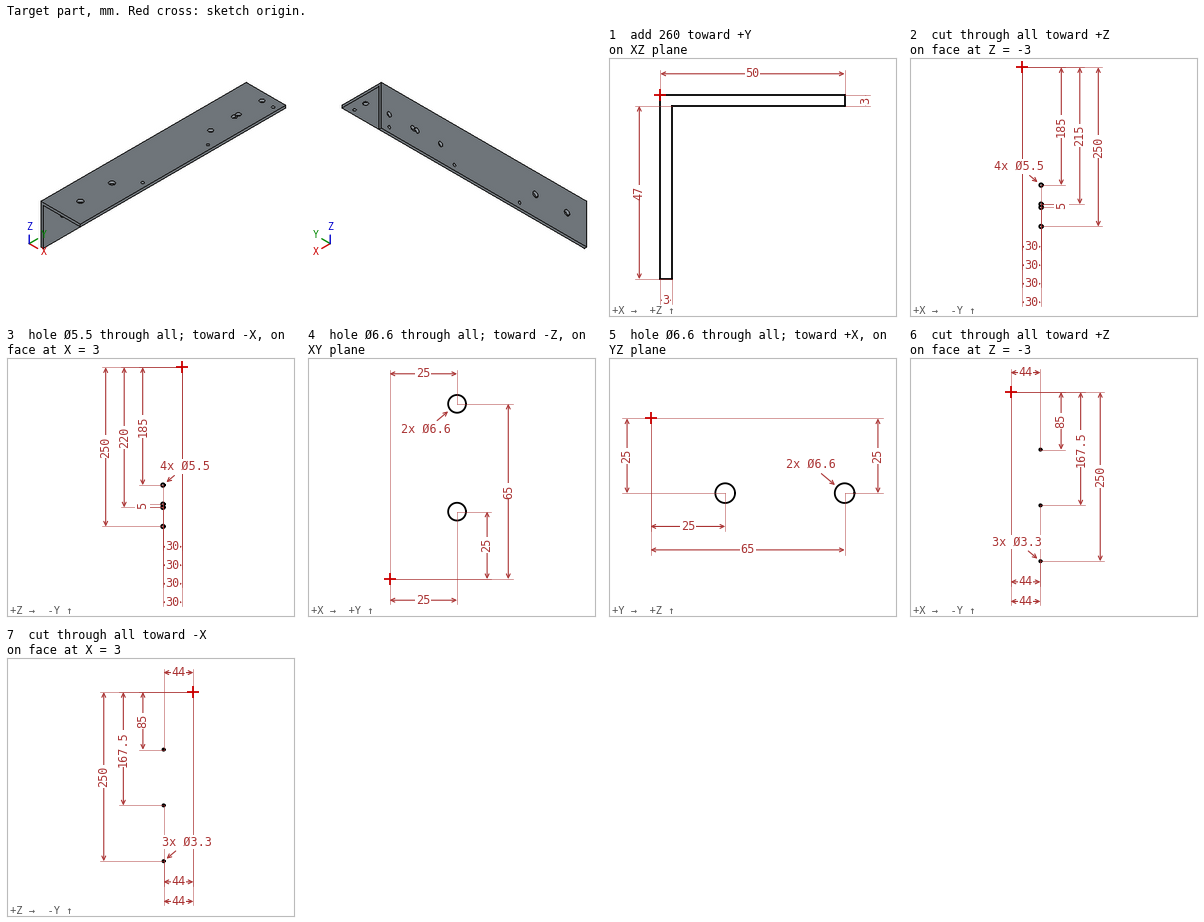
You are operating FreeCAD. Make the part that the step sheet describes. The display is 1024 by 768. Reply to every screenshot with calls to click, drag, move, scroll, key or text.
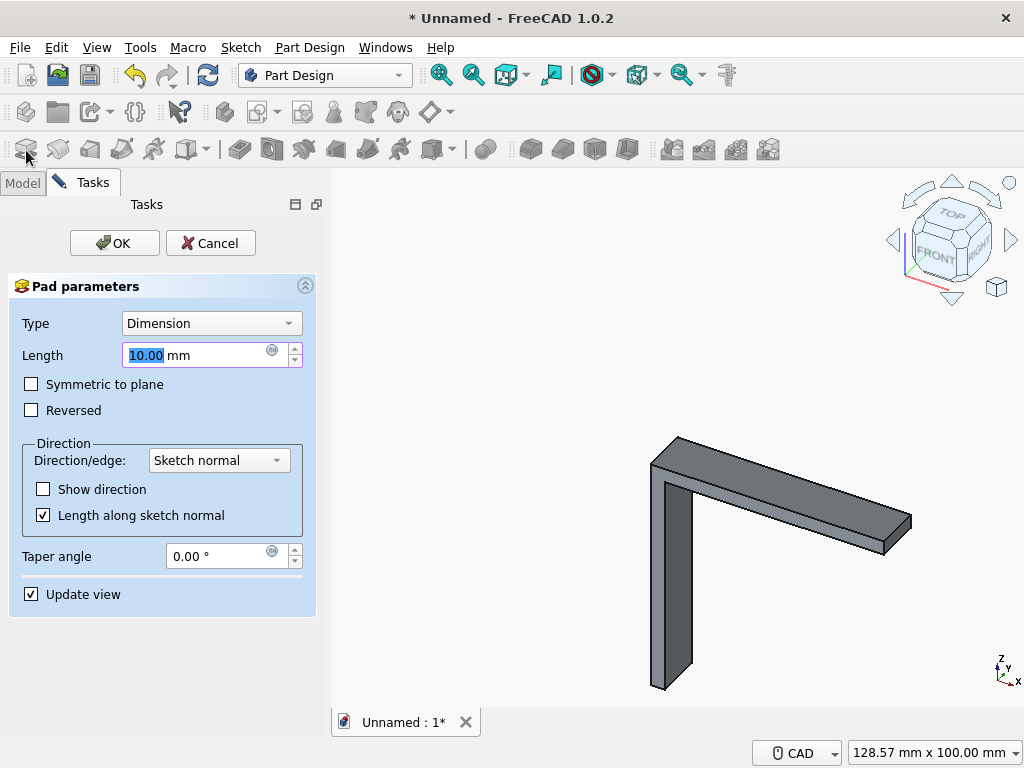
text(260)
key(Tab)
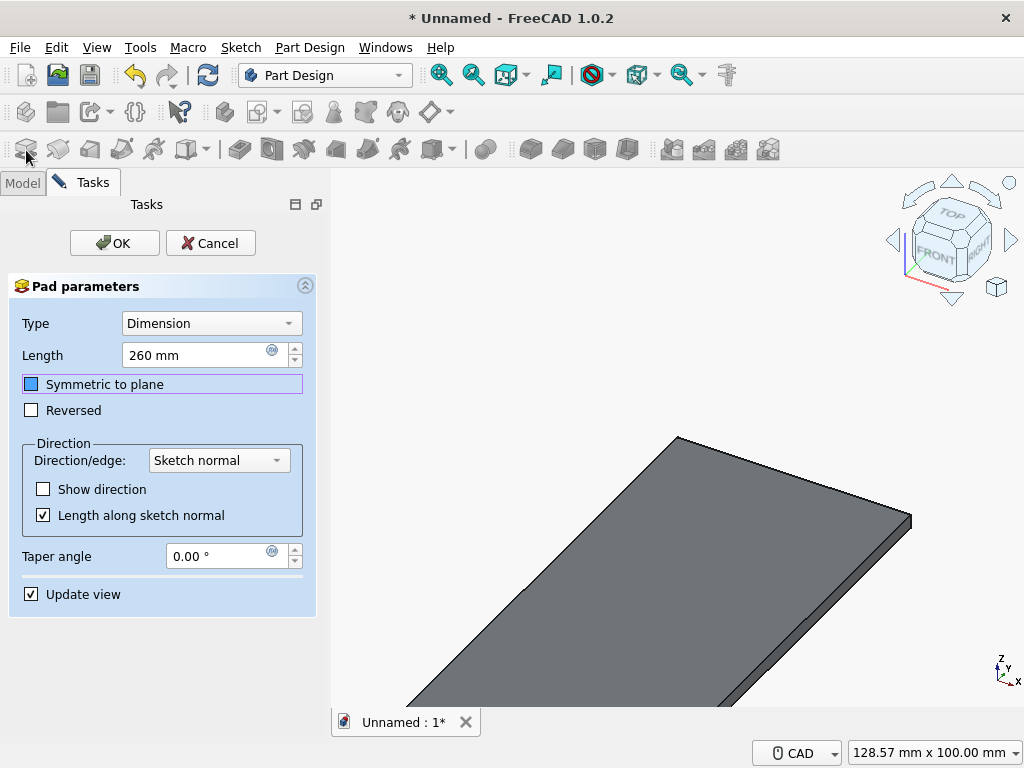
click(30, 410)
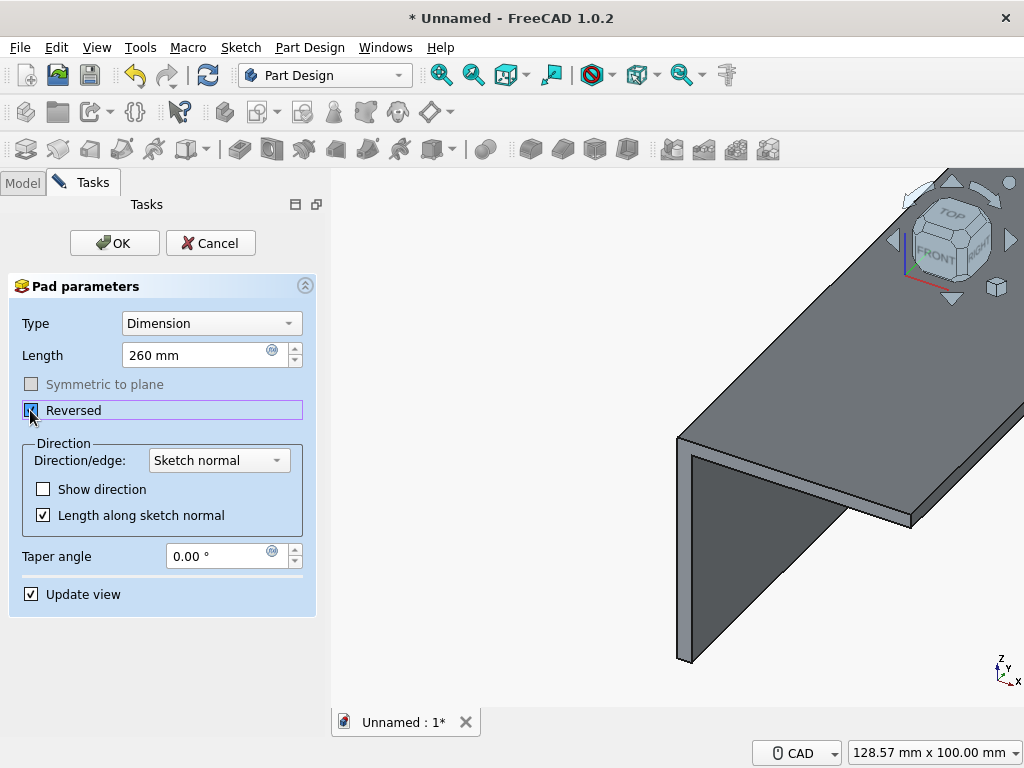
click(115, 243)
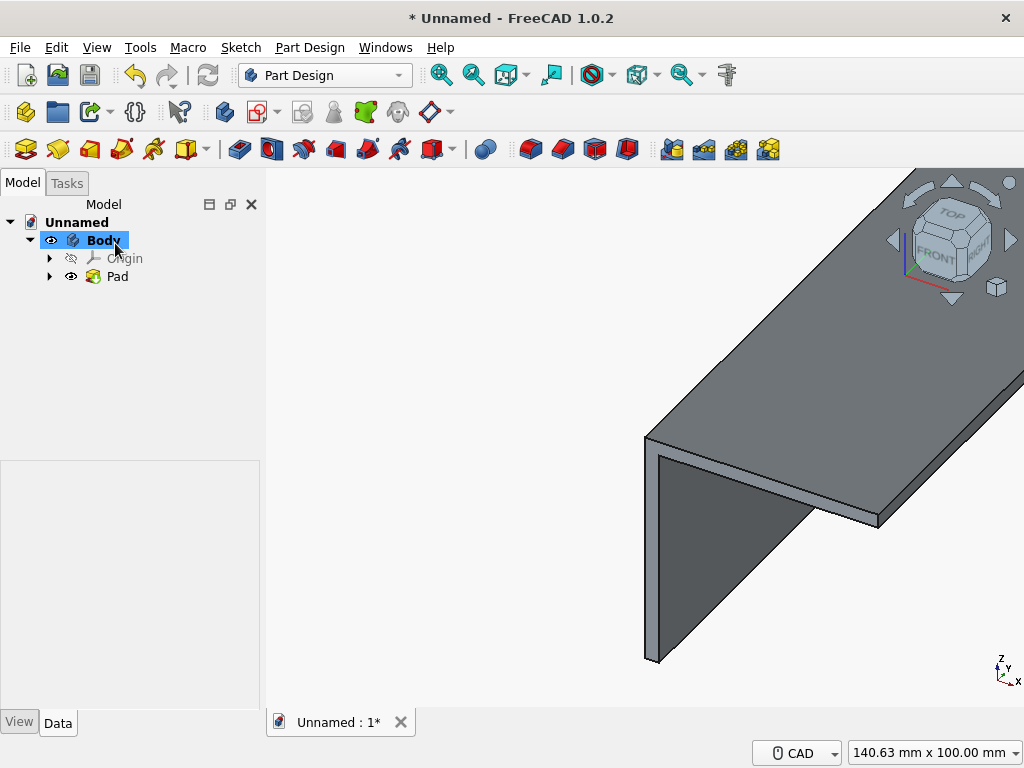
key(v)
key(f)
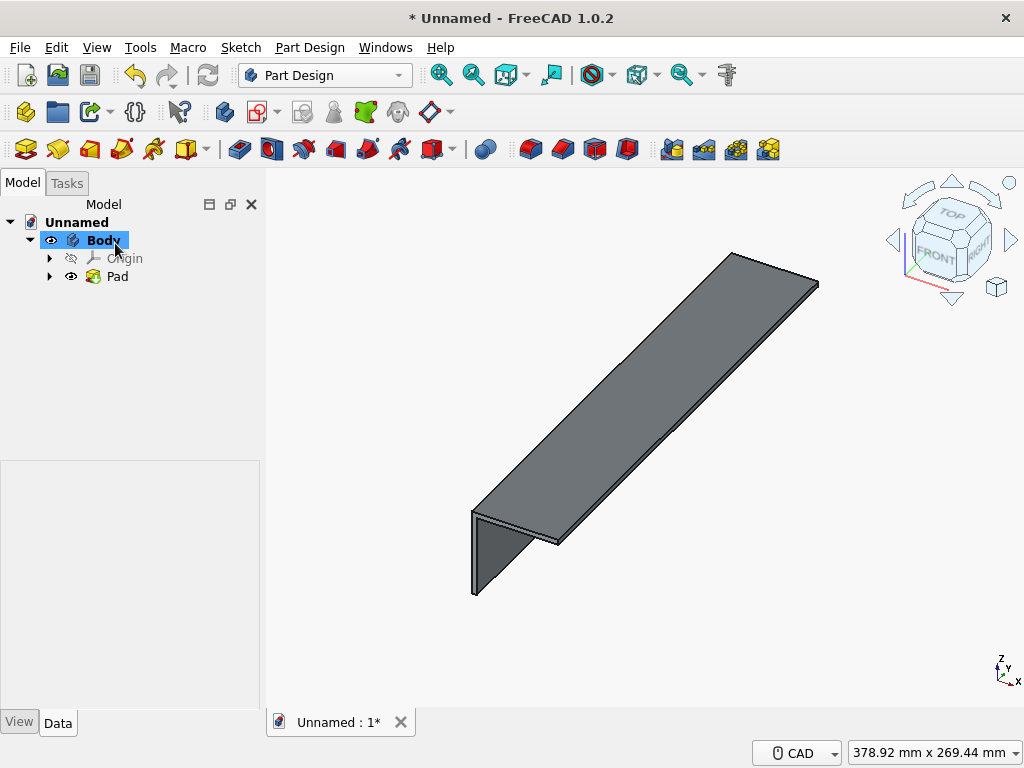
key(5)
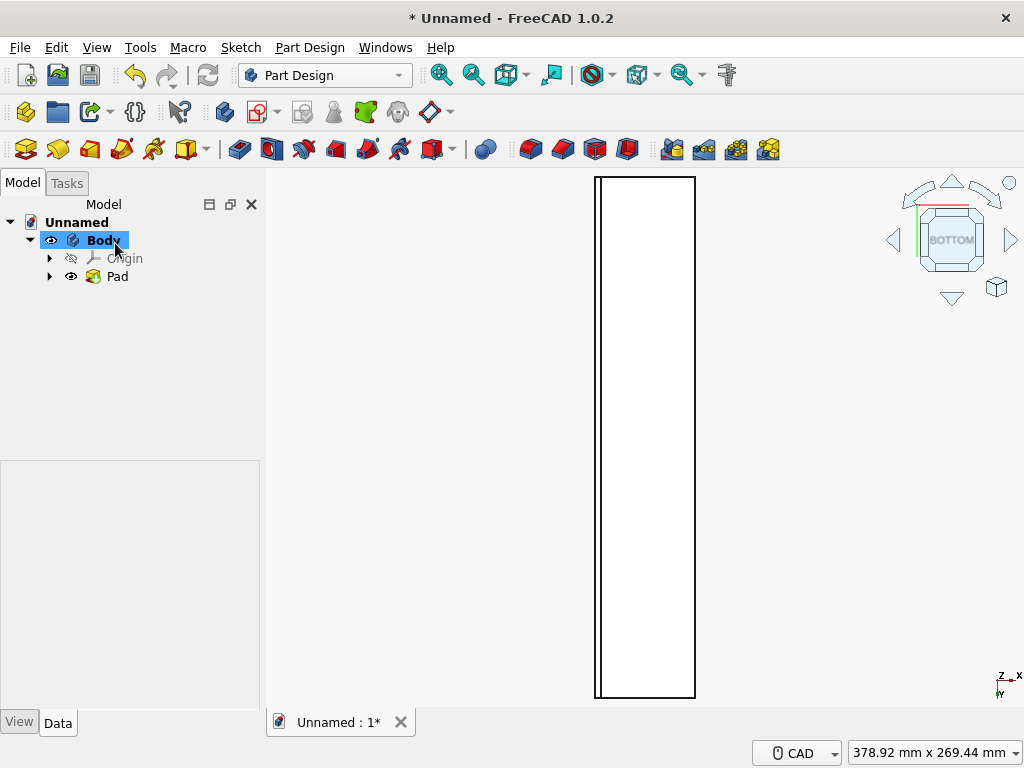
click(648, 585)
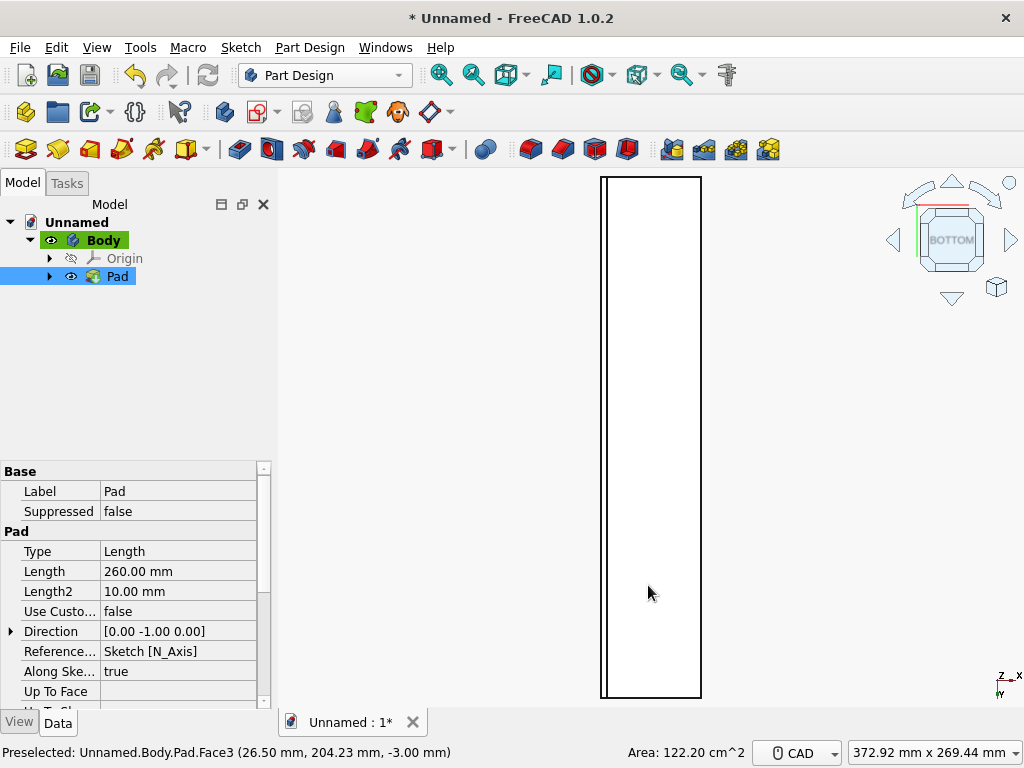
click(258, 112)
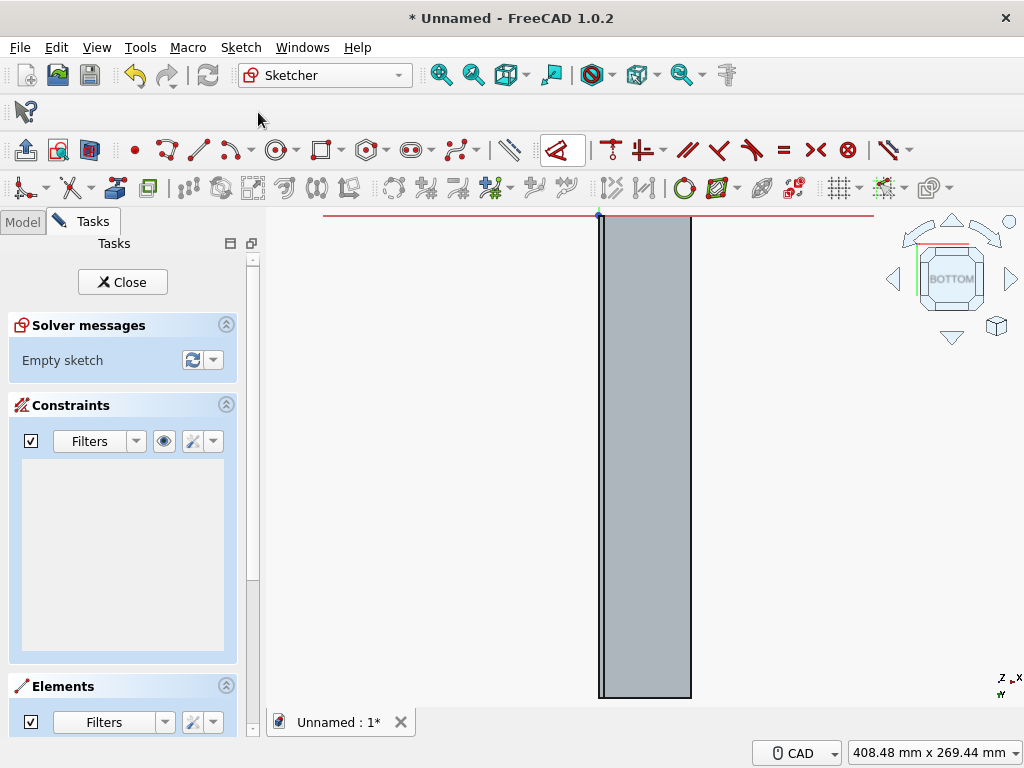
key(q)
key(s)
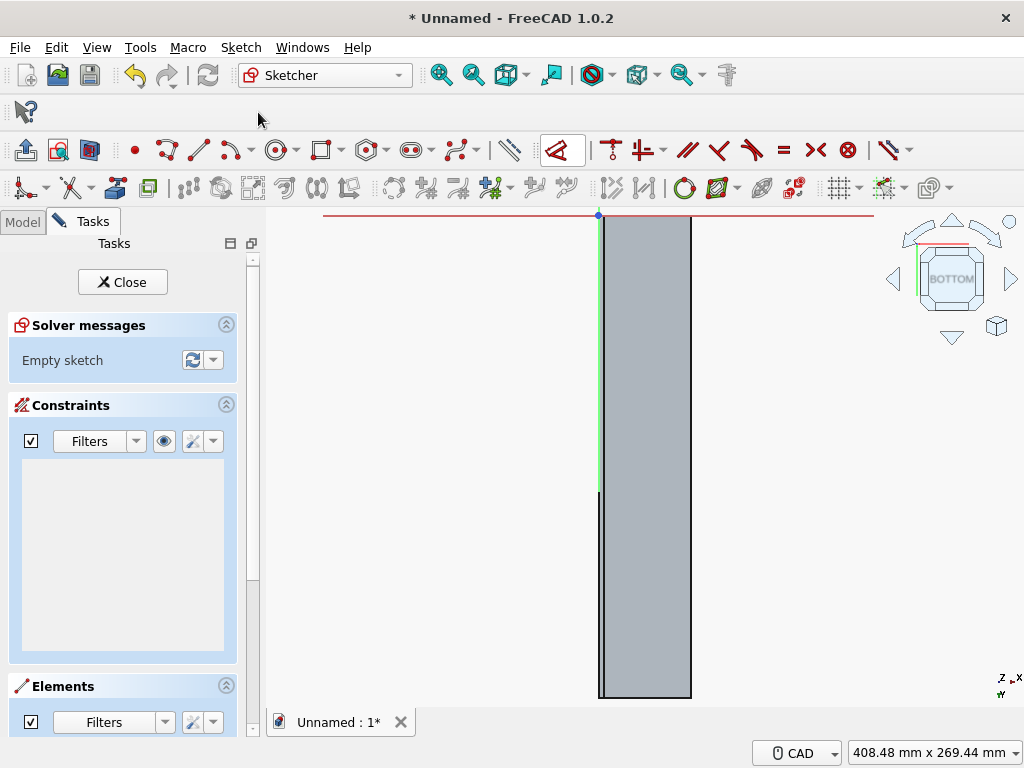
scroll(576, 457, down, 5)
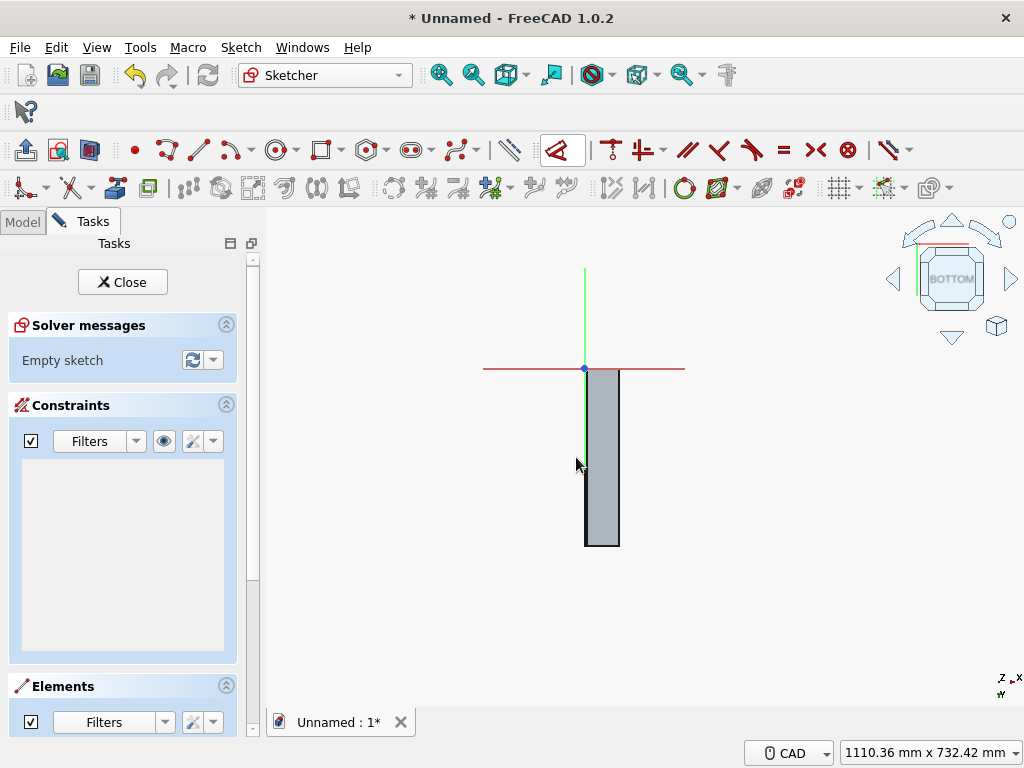
scroll(611, 529, up, 9)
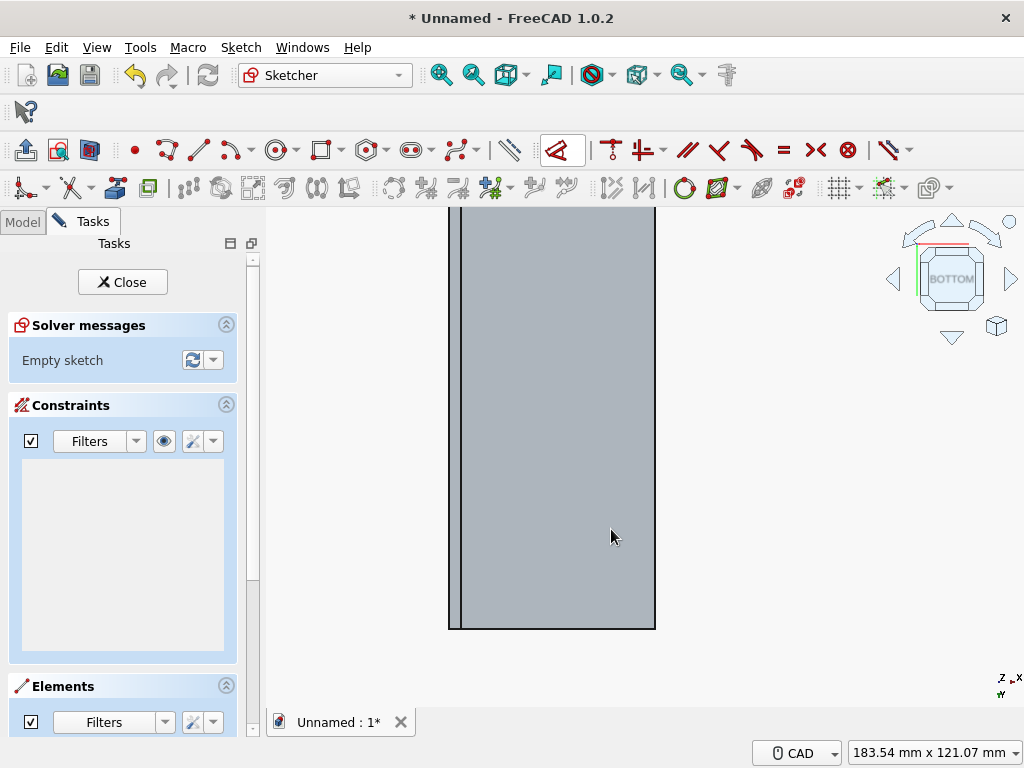
key(g)
key(c)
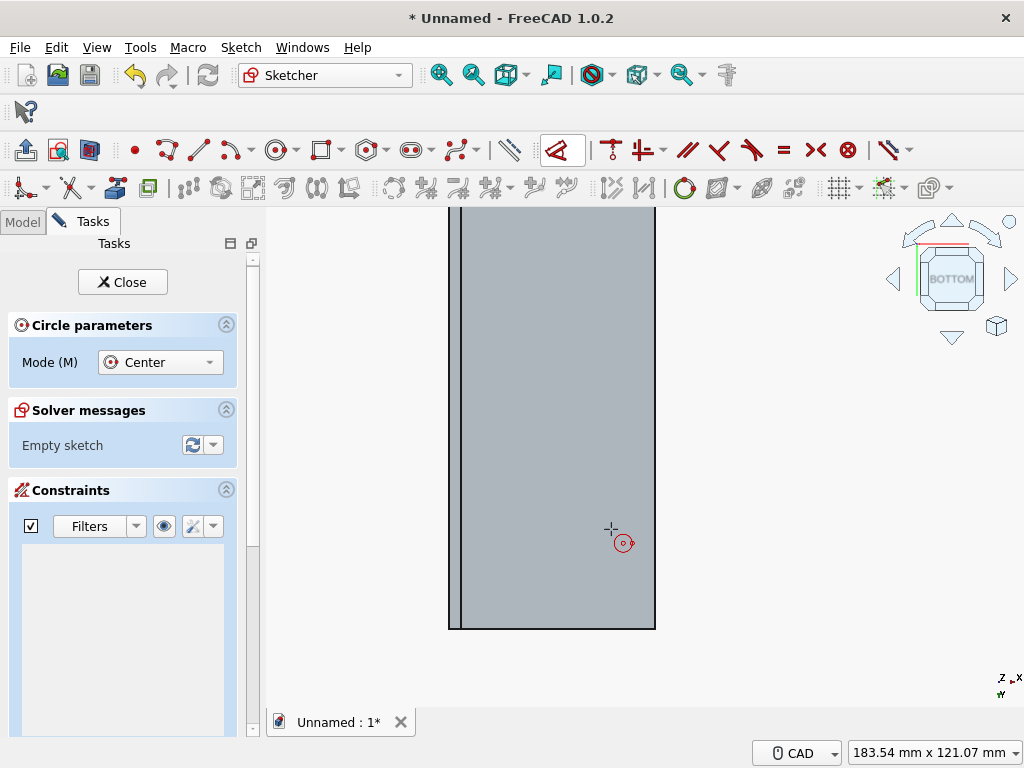
scroll(573, 588, up, 4)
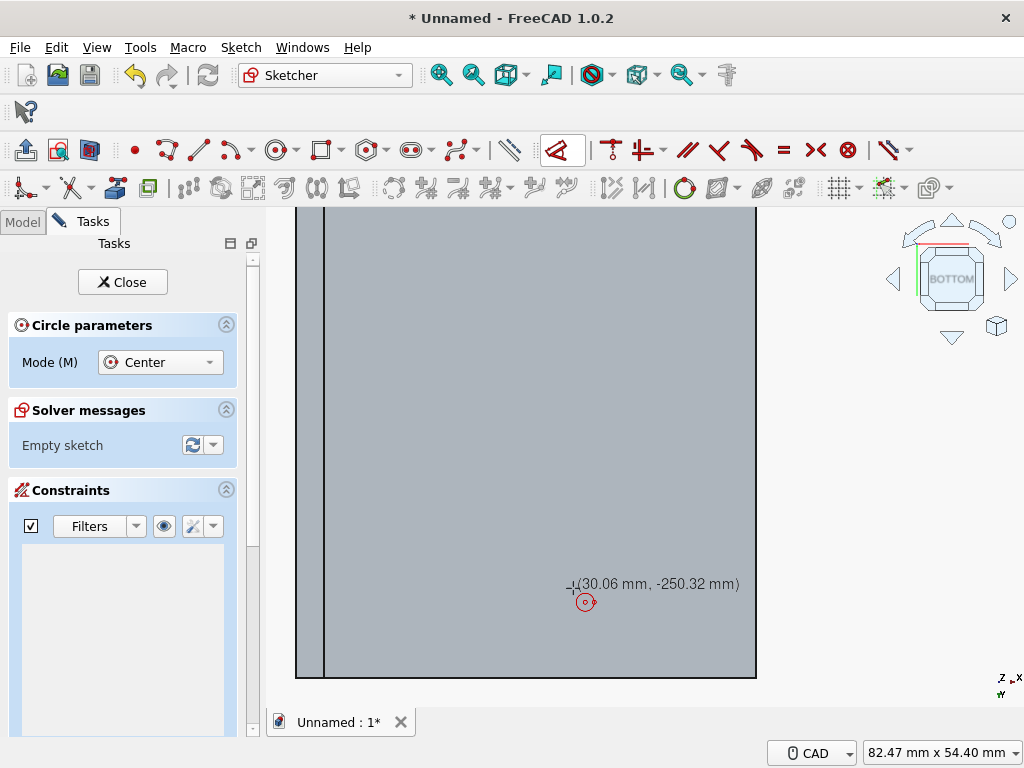
click(572, 586)
click(590, 568)